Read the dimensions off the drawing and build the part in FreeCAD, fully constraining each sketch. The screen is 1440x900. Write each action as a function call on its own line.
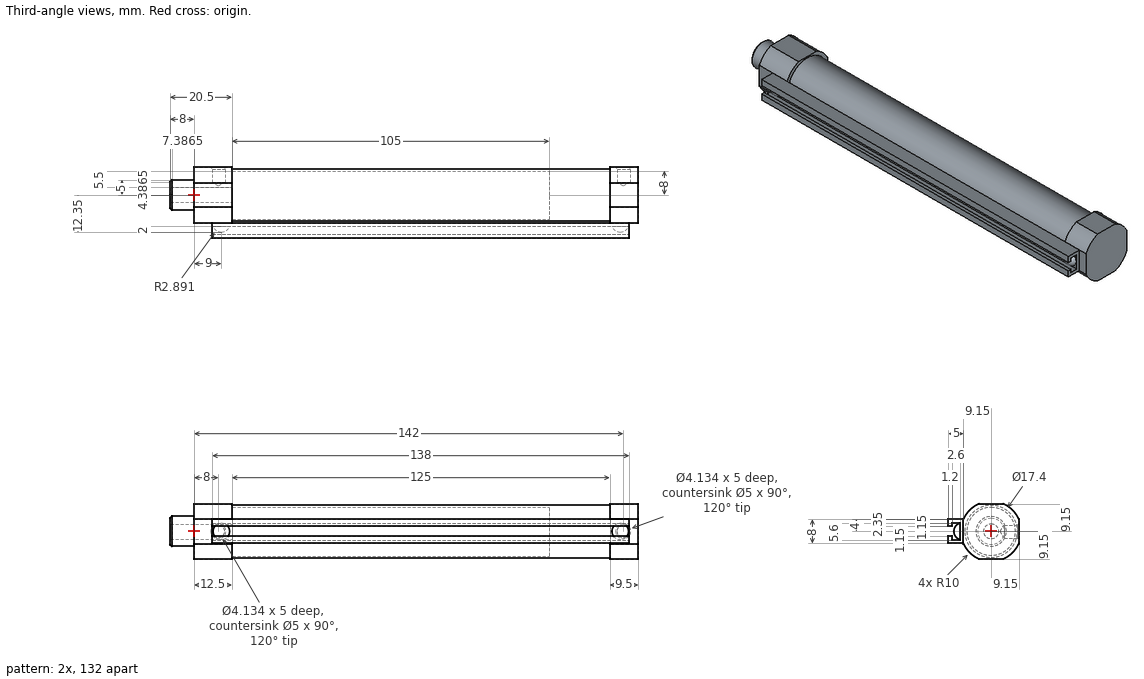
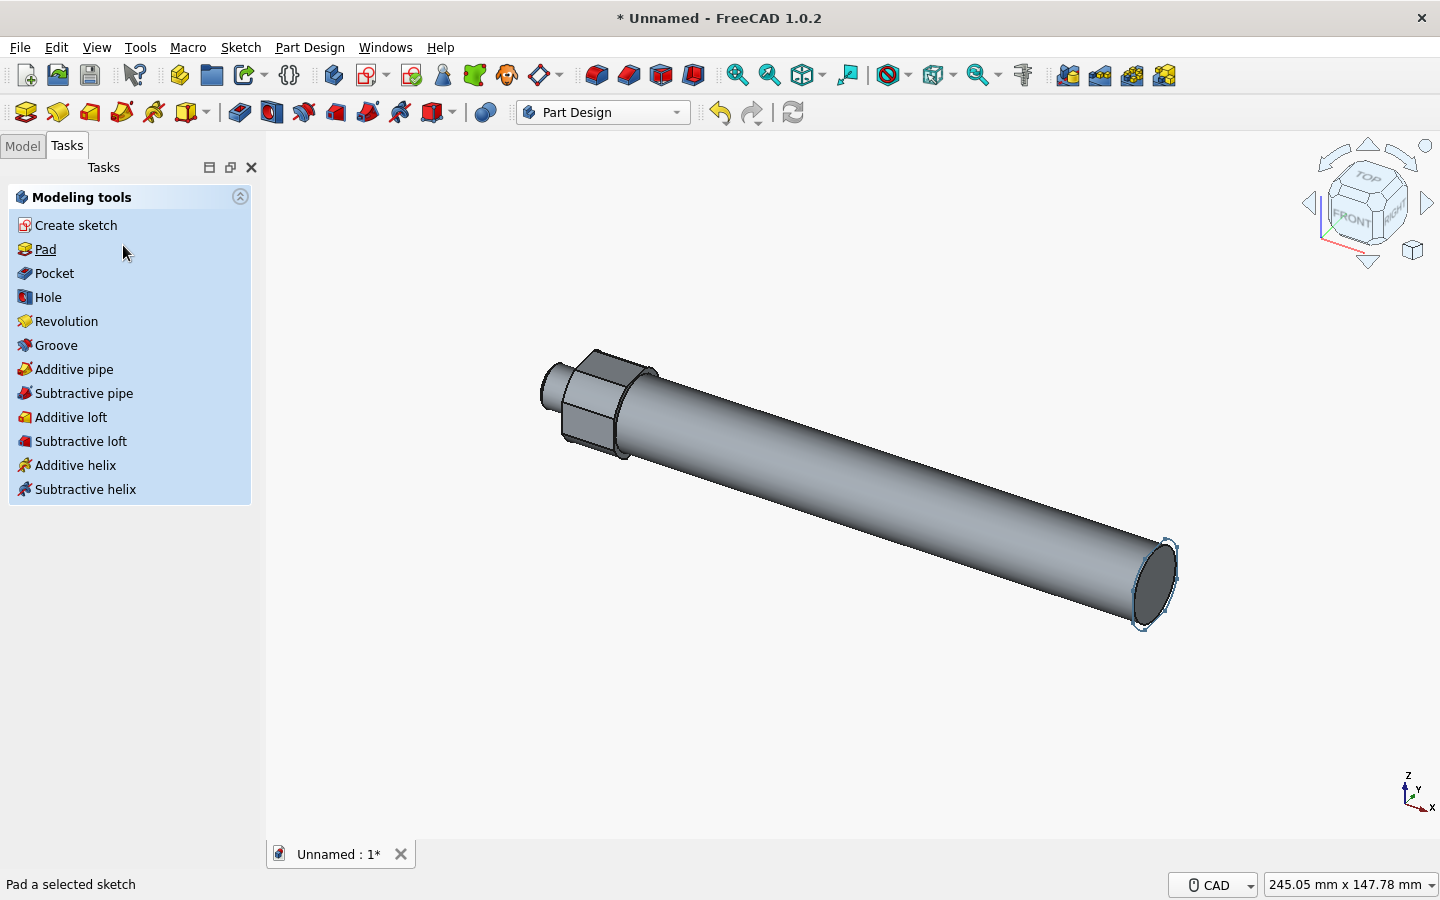
click(26, 112)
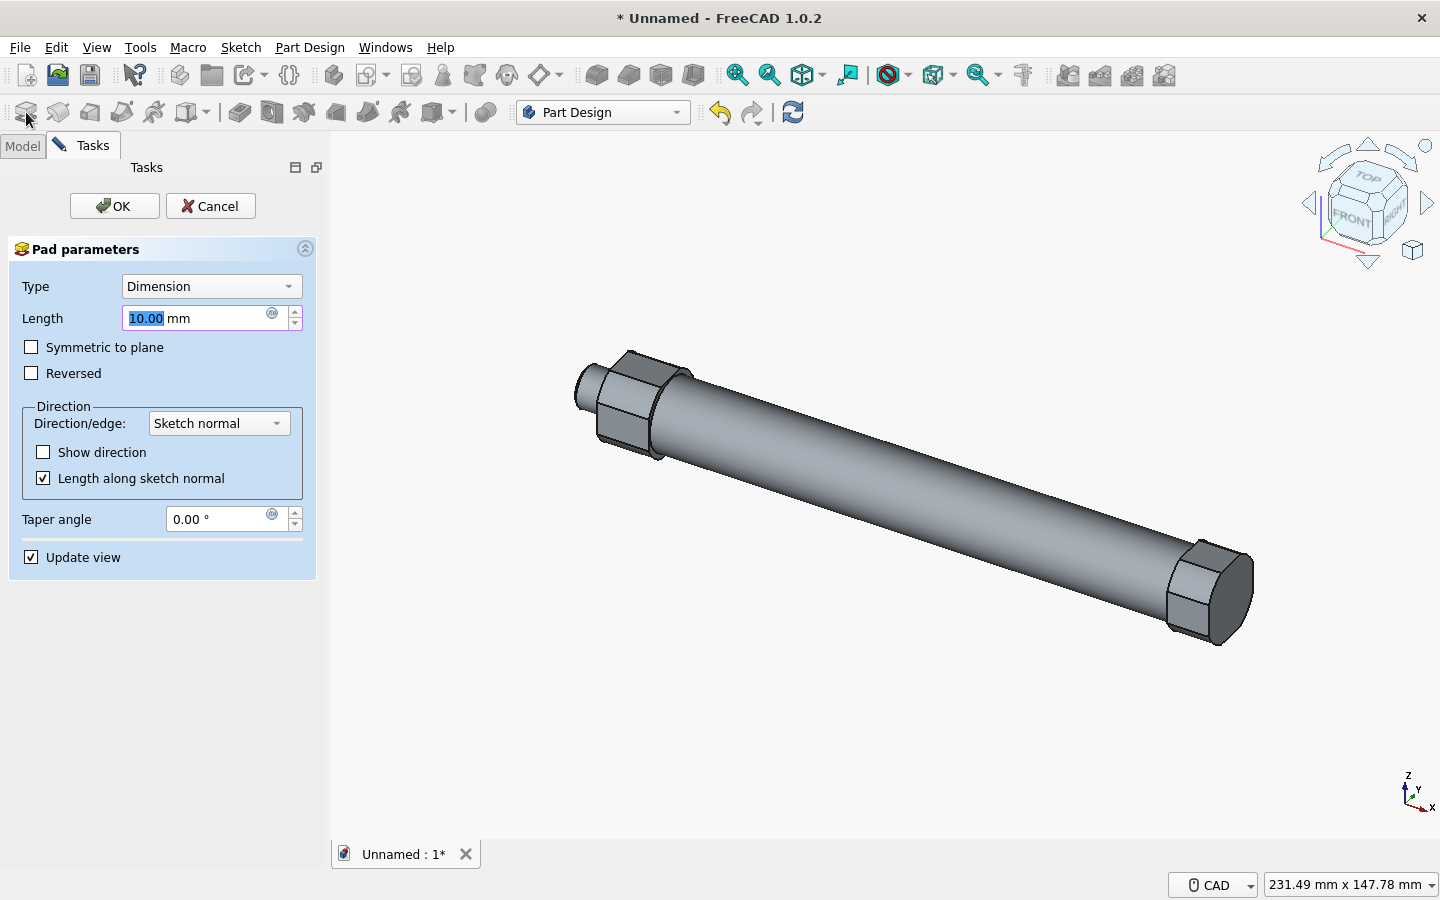
text(9.5)
key(Tab)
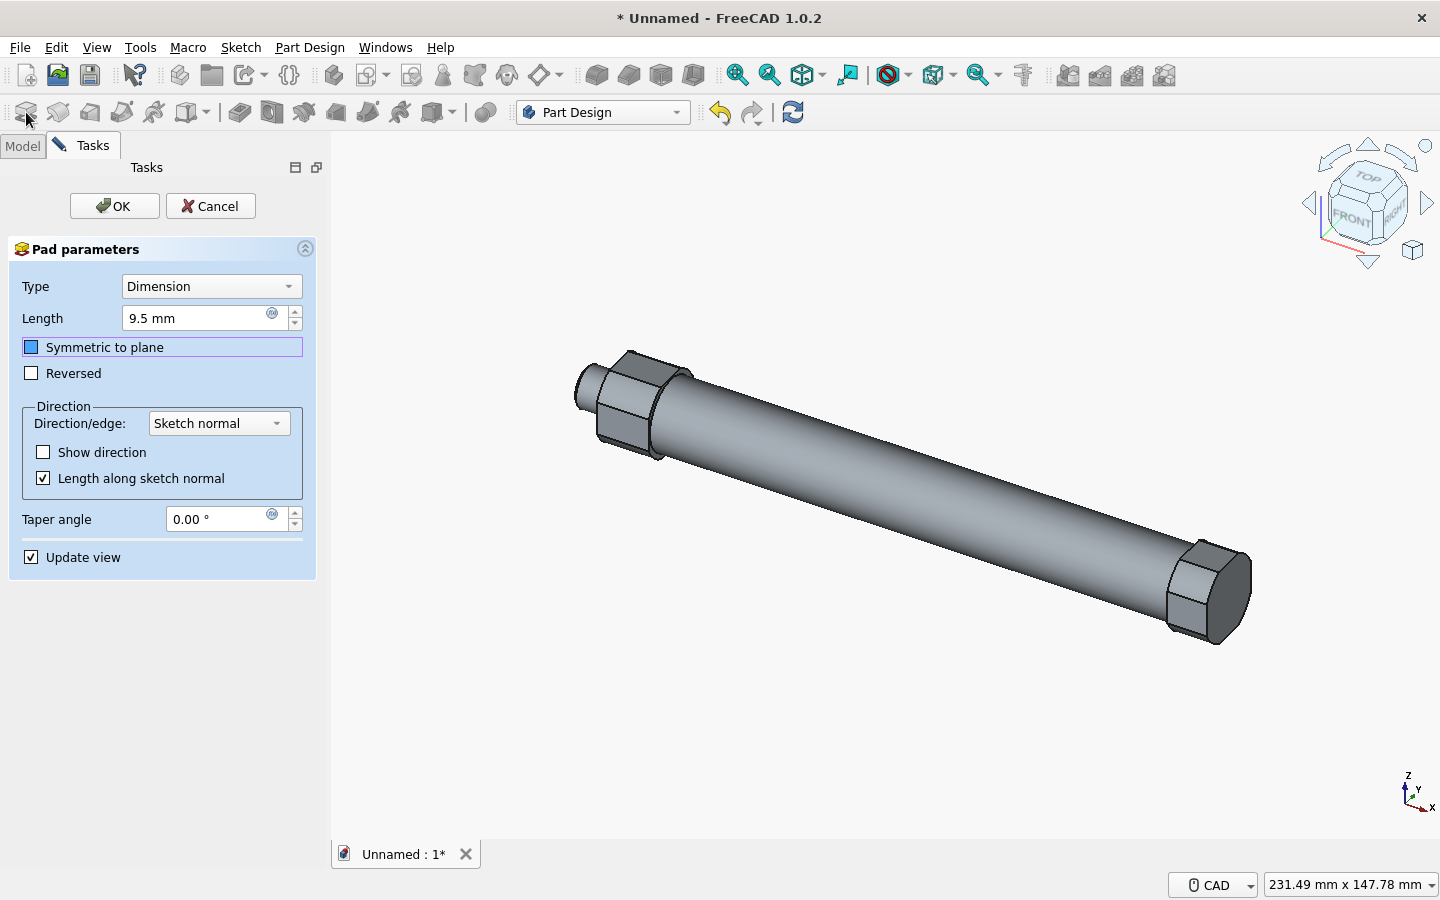
click(115, 206)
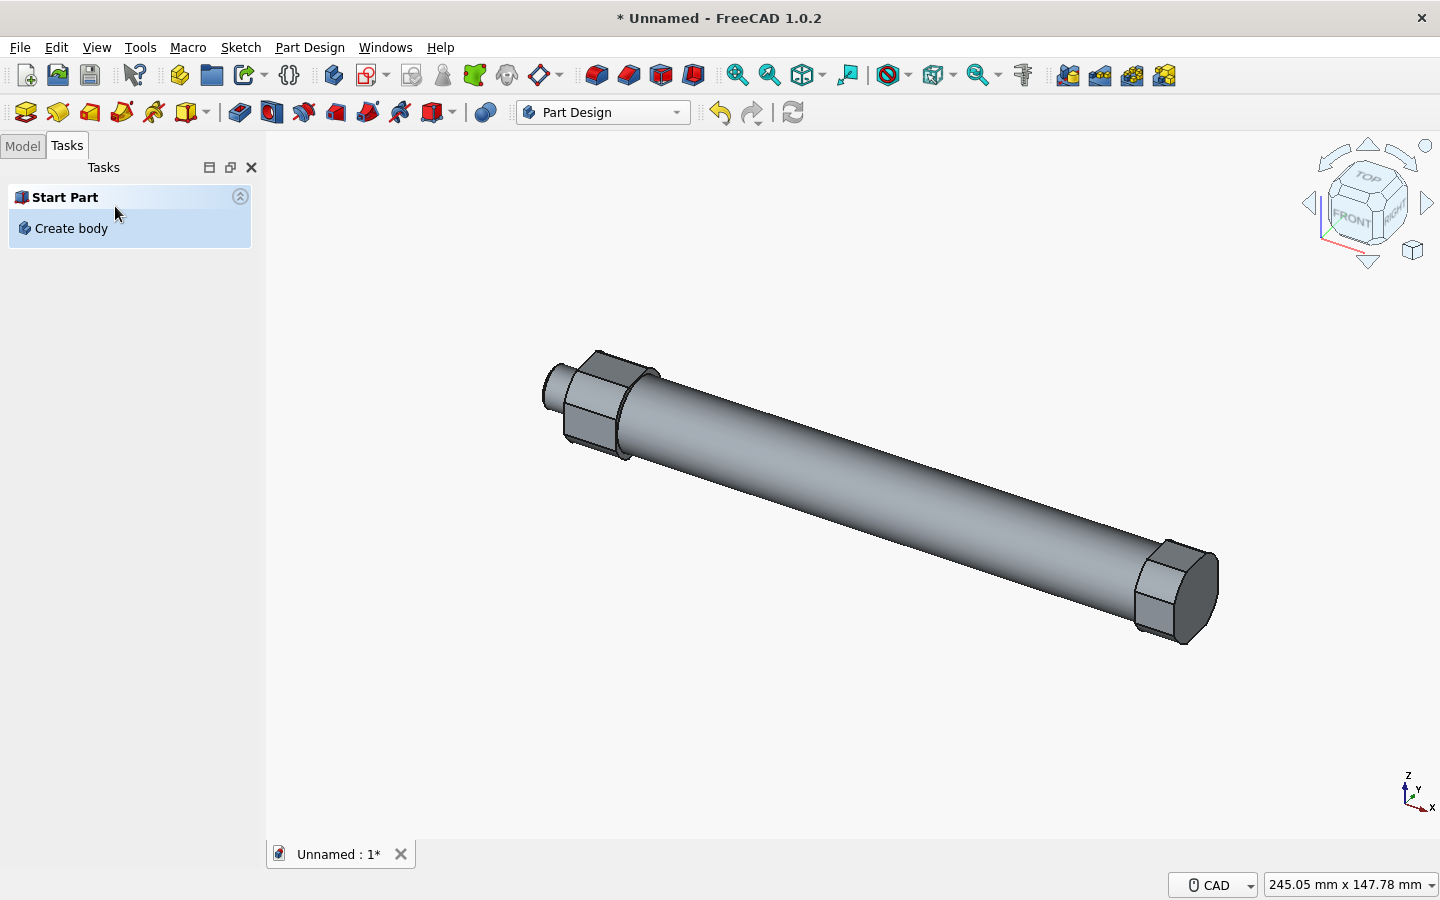
key(4)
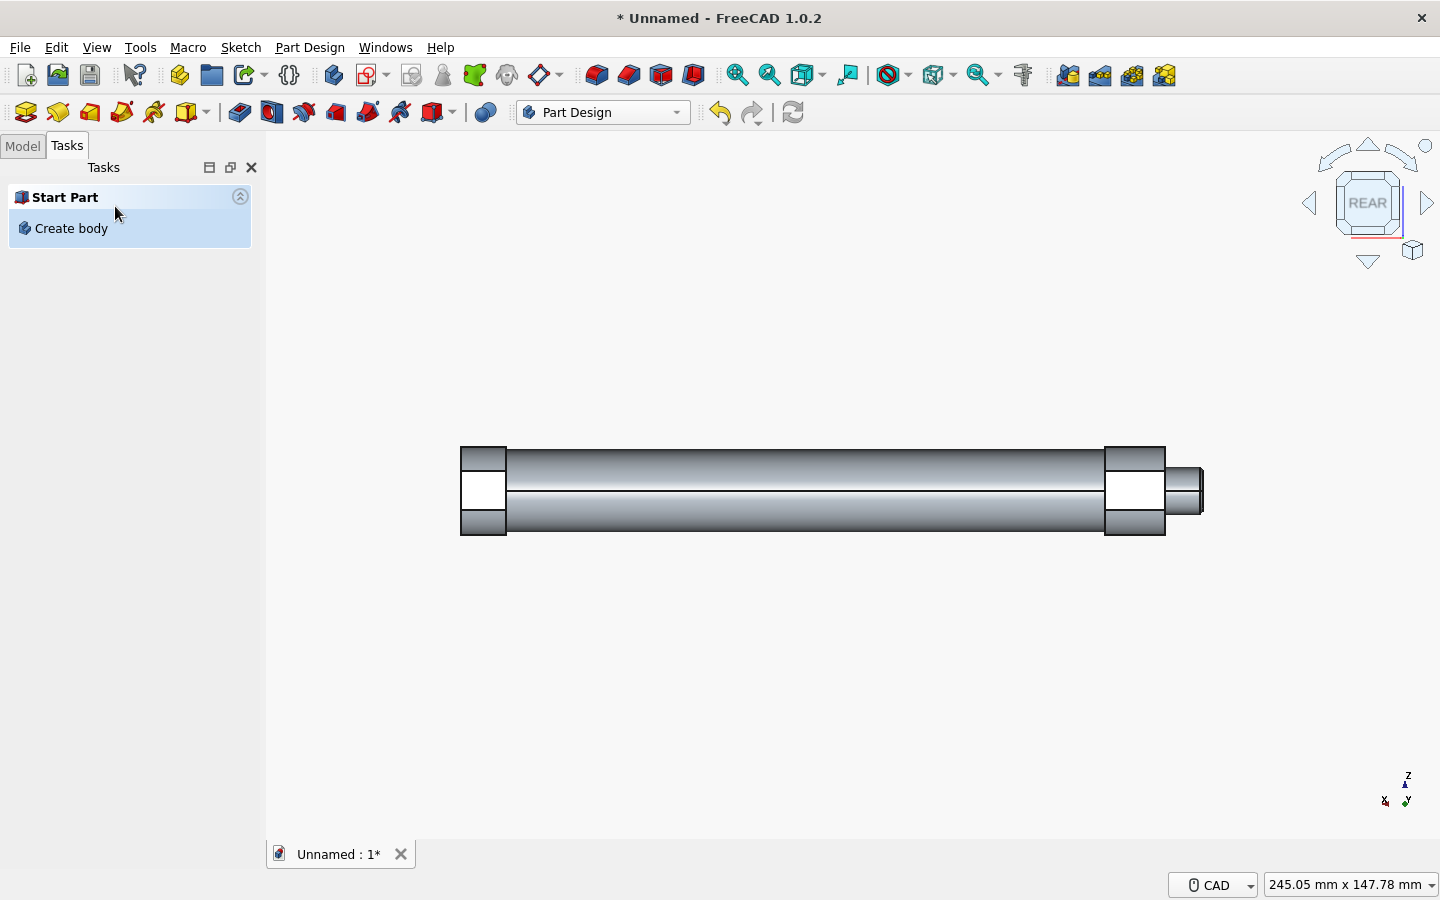
click(1127, 490)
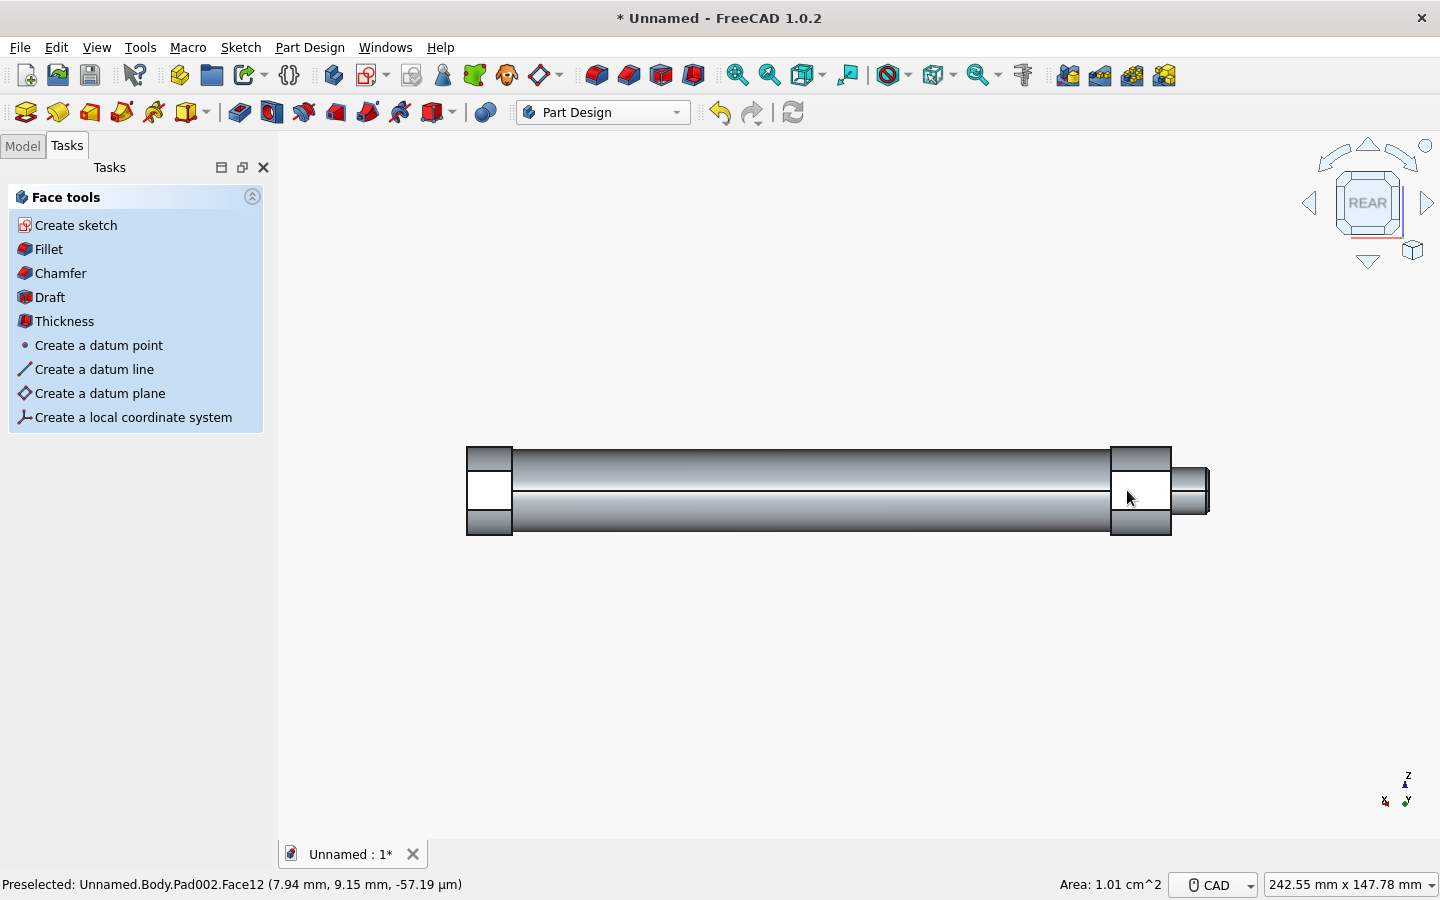
click(366, 76)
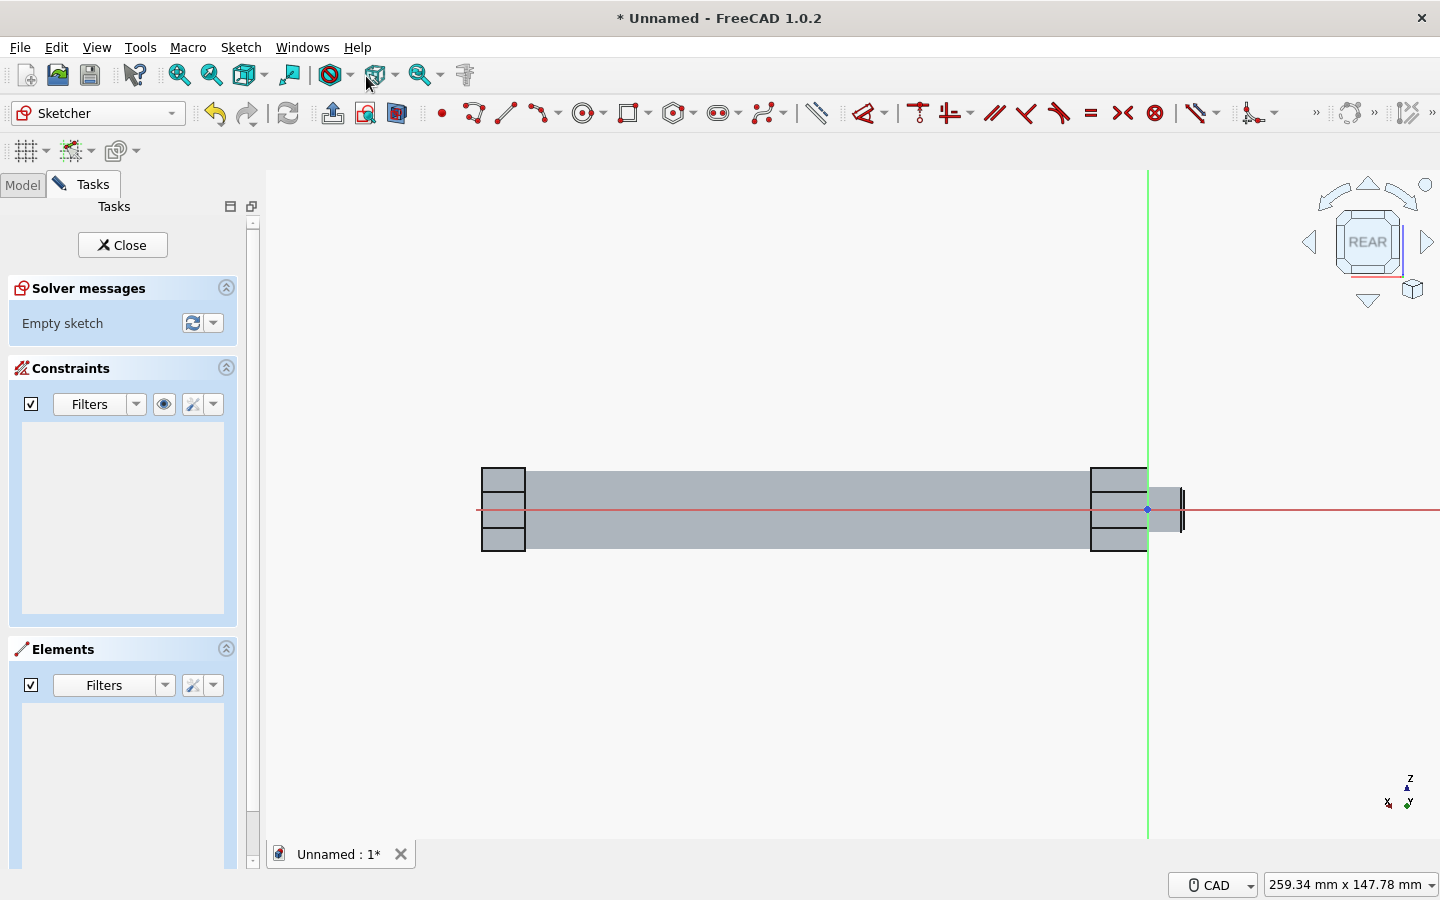
scroll(1147, 510, up, 14)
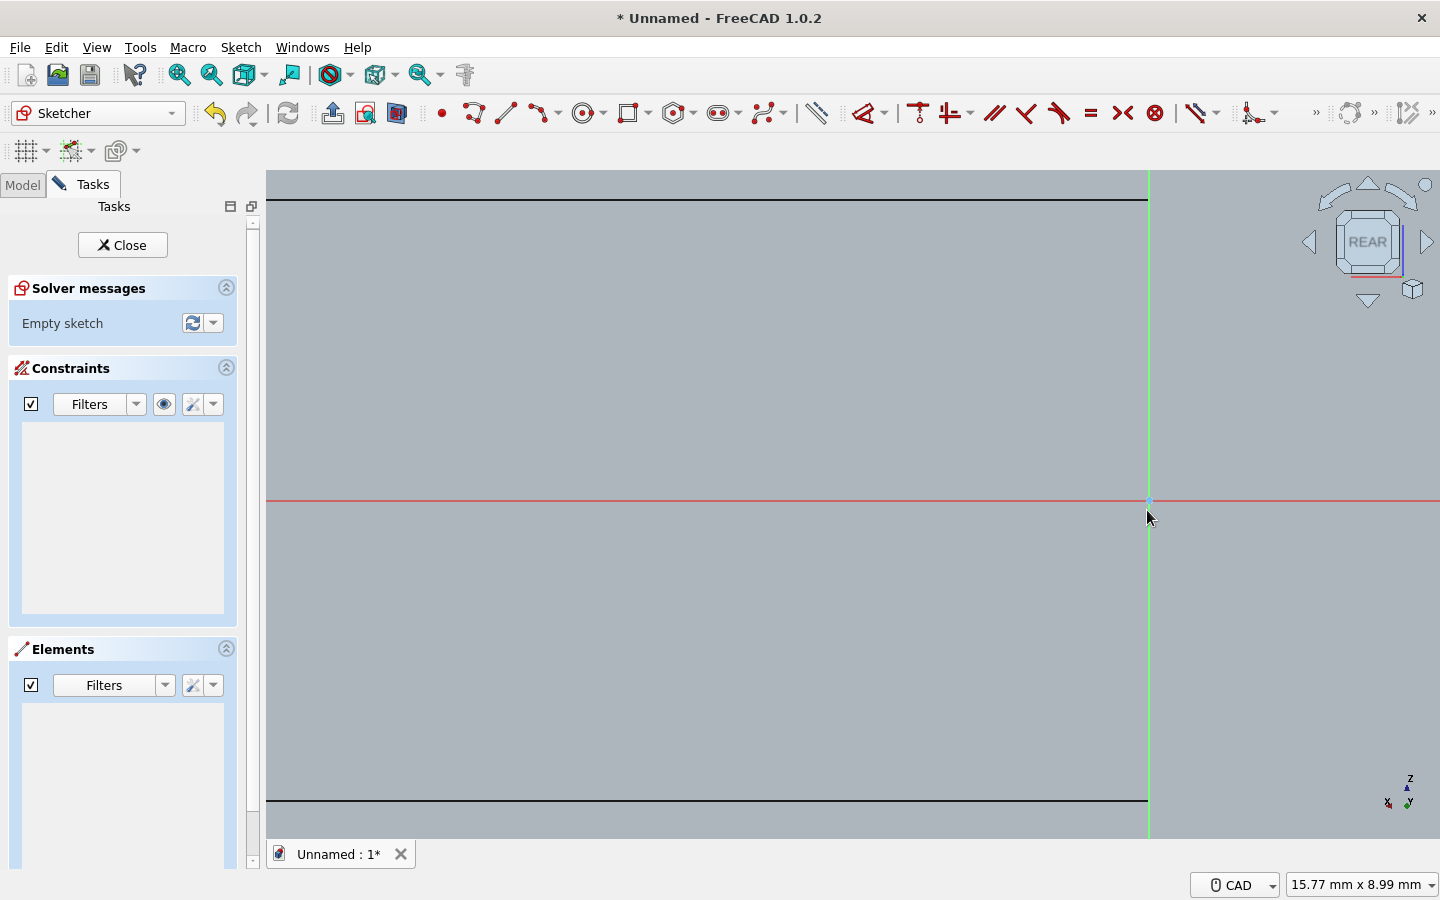
click(584, 114)